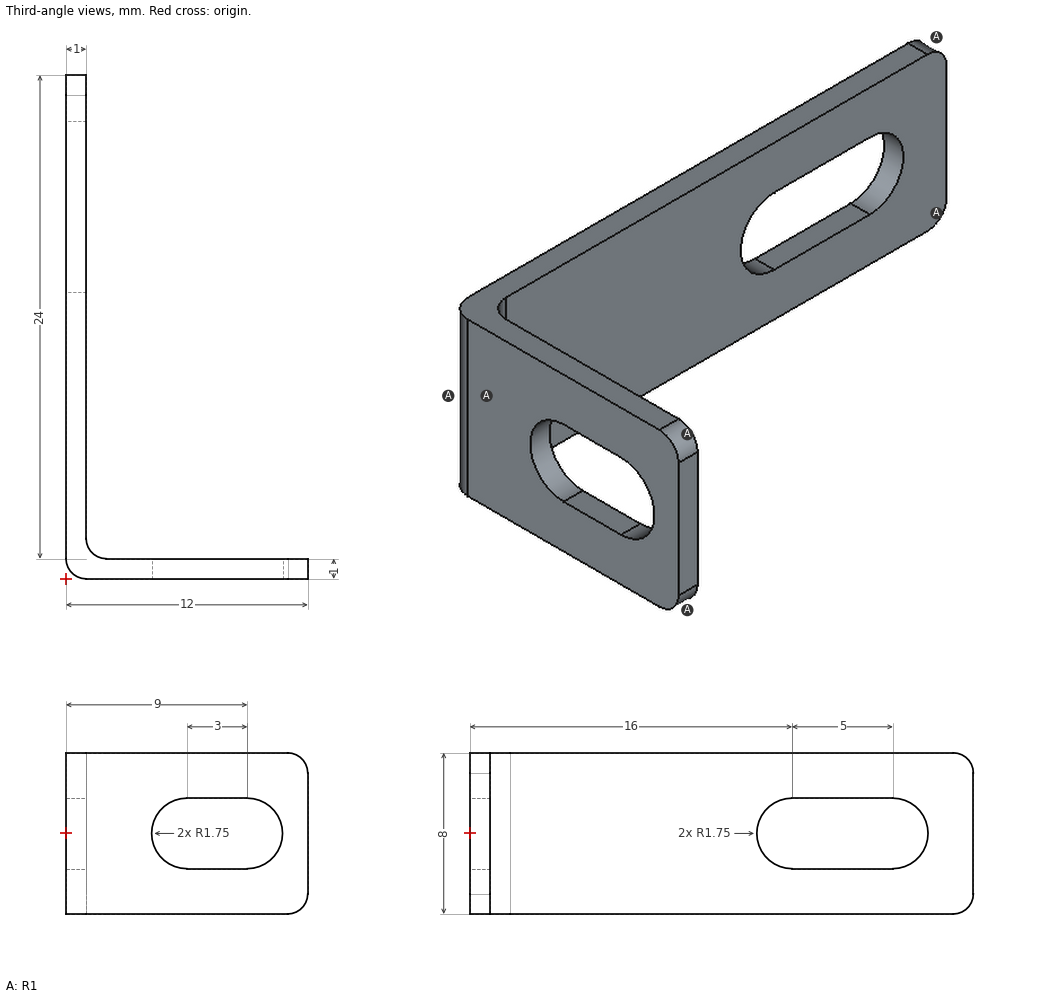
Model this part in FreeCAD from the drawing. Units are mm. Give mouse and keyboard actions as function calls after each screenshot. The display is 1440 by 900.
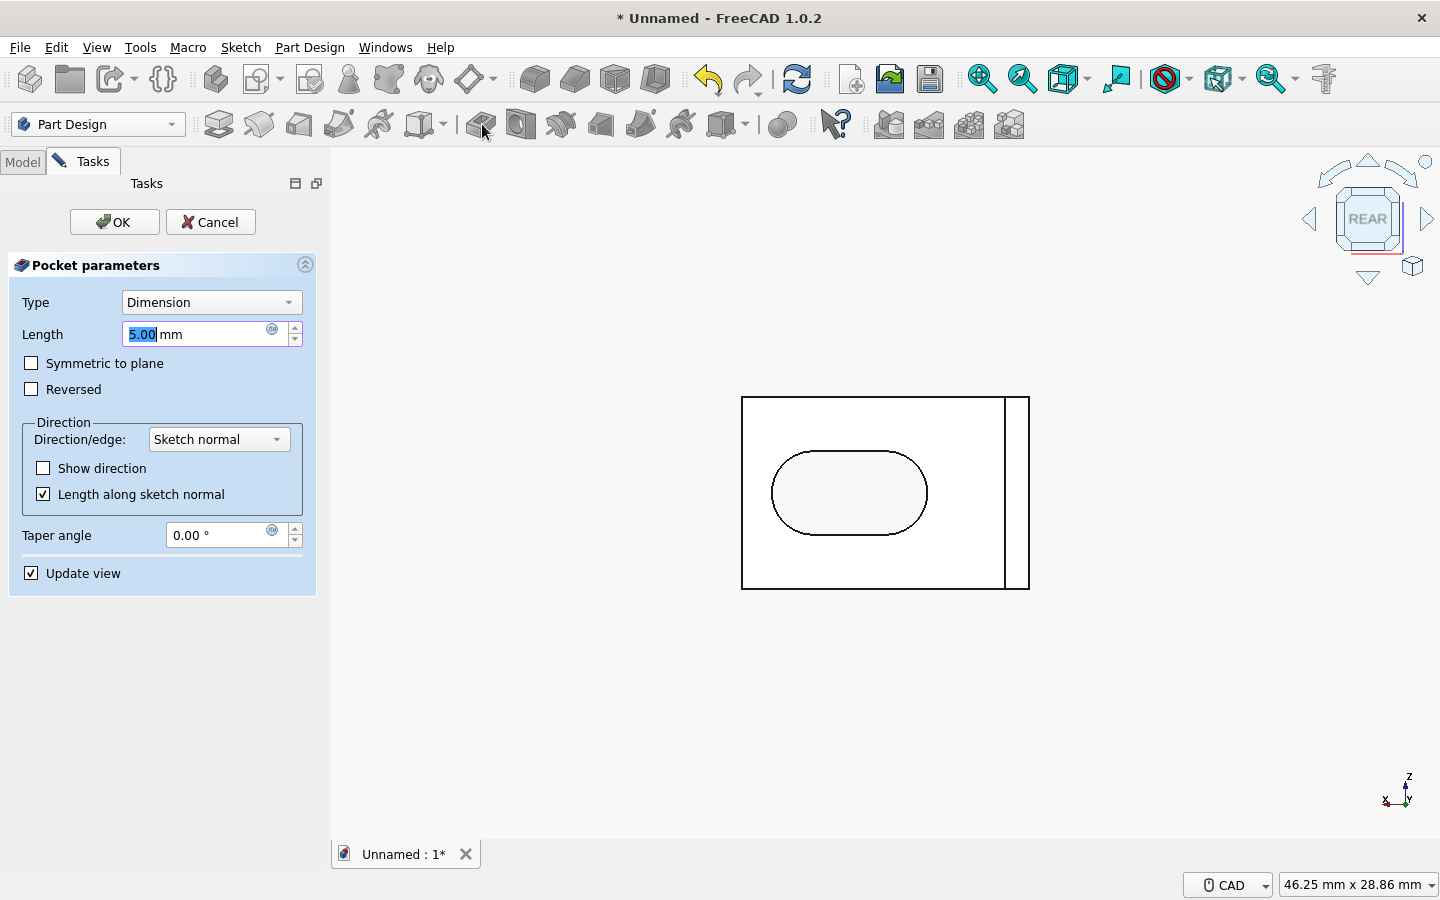
click(212, 302)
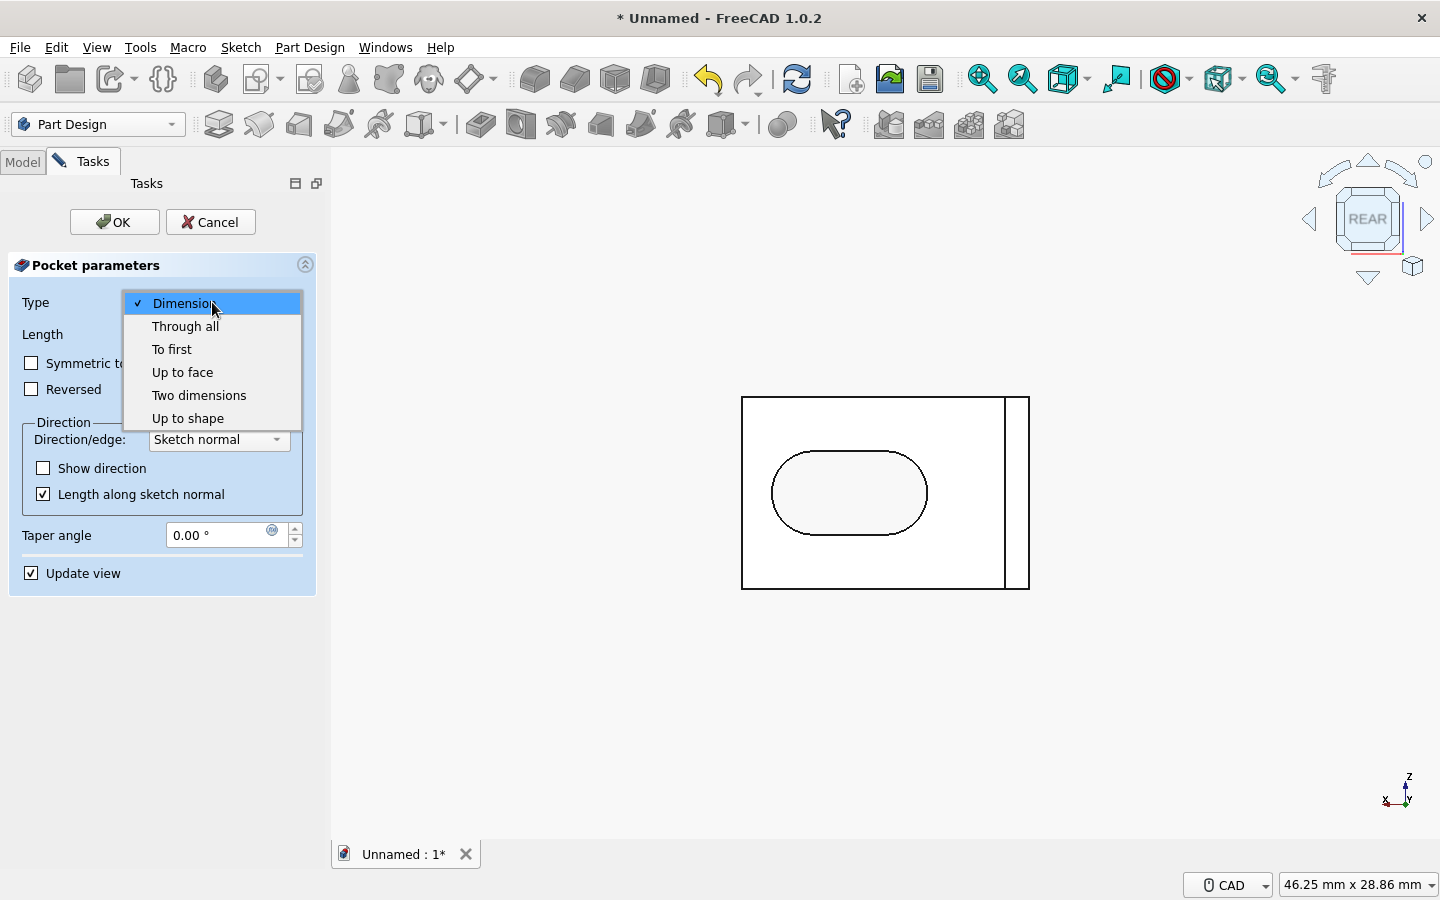
click(212, 326)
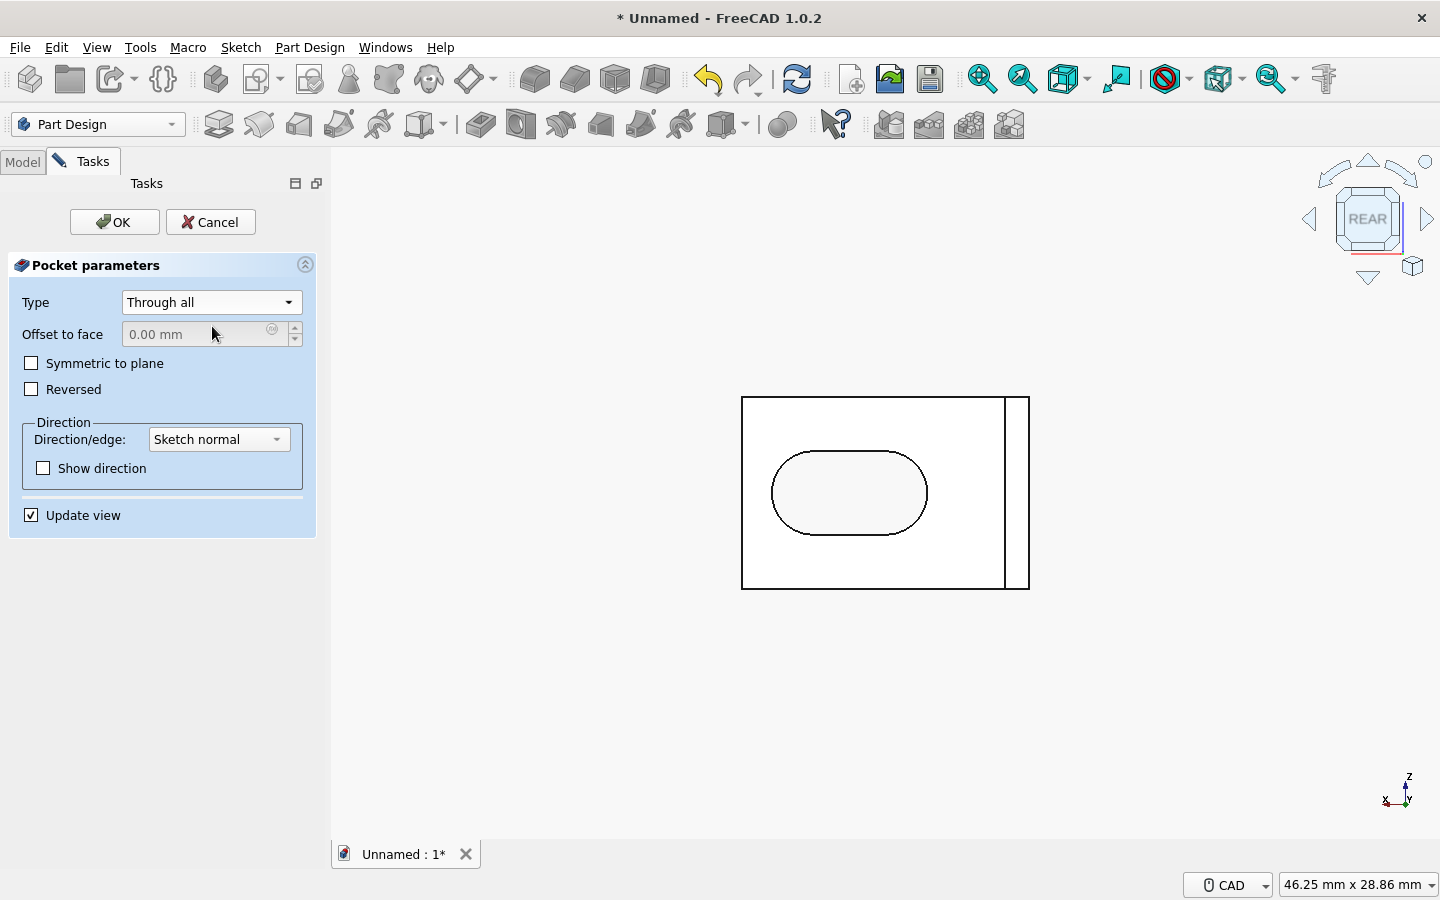
click(30, 389)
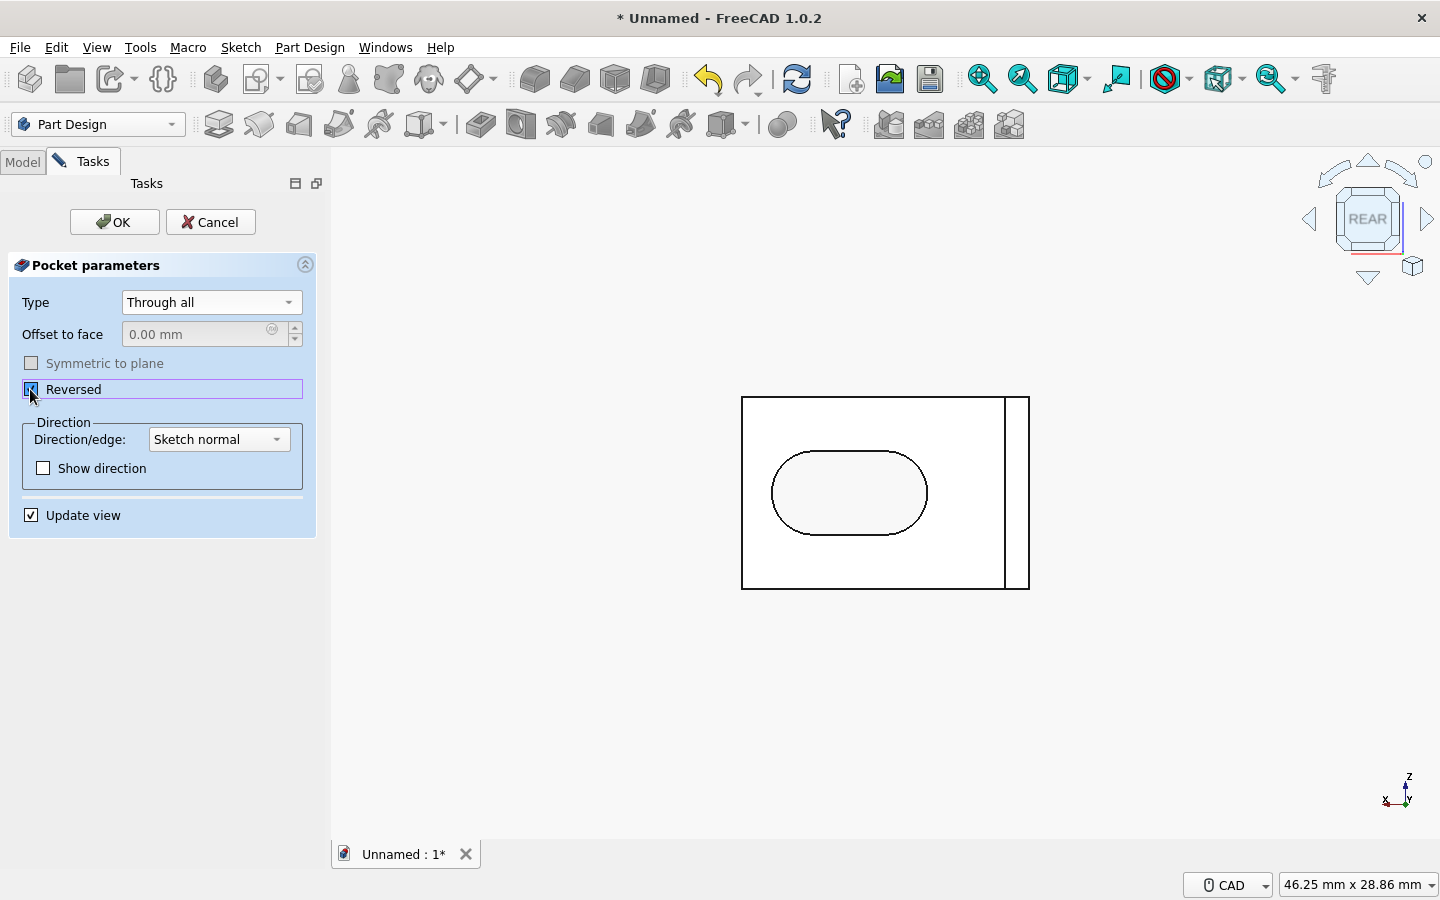
click(115, 222)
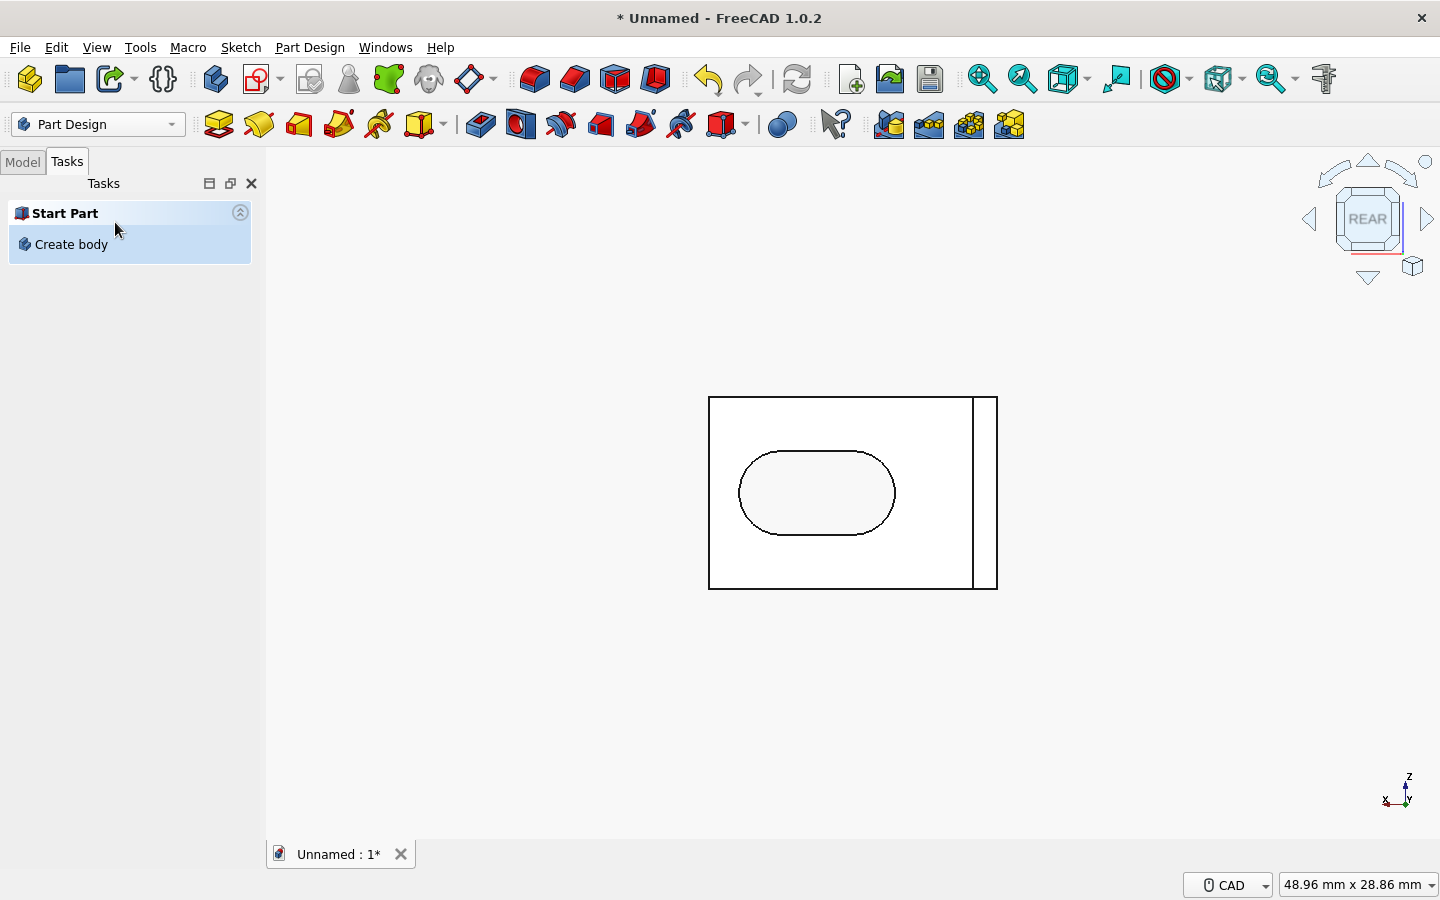
key(v)
key(f)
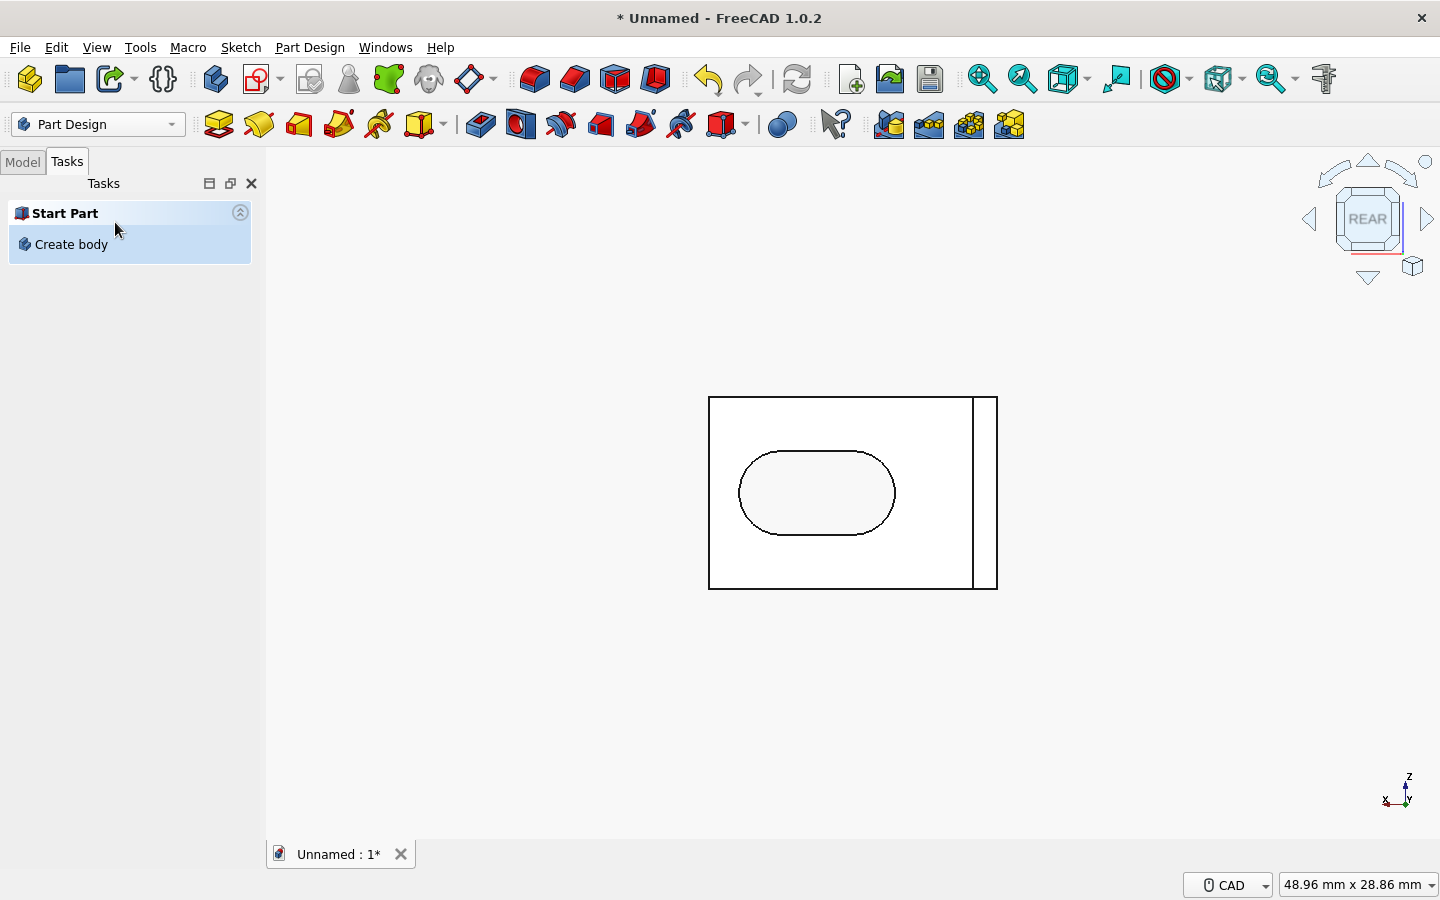
click(985, 396)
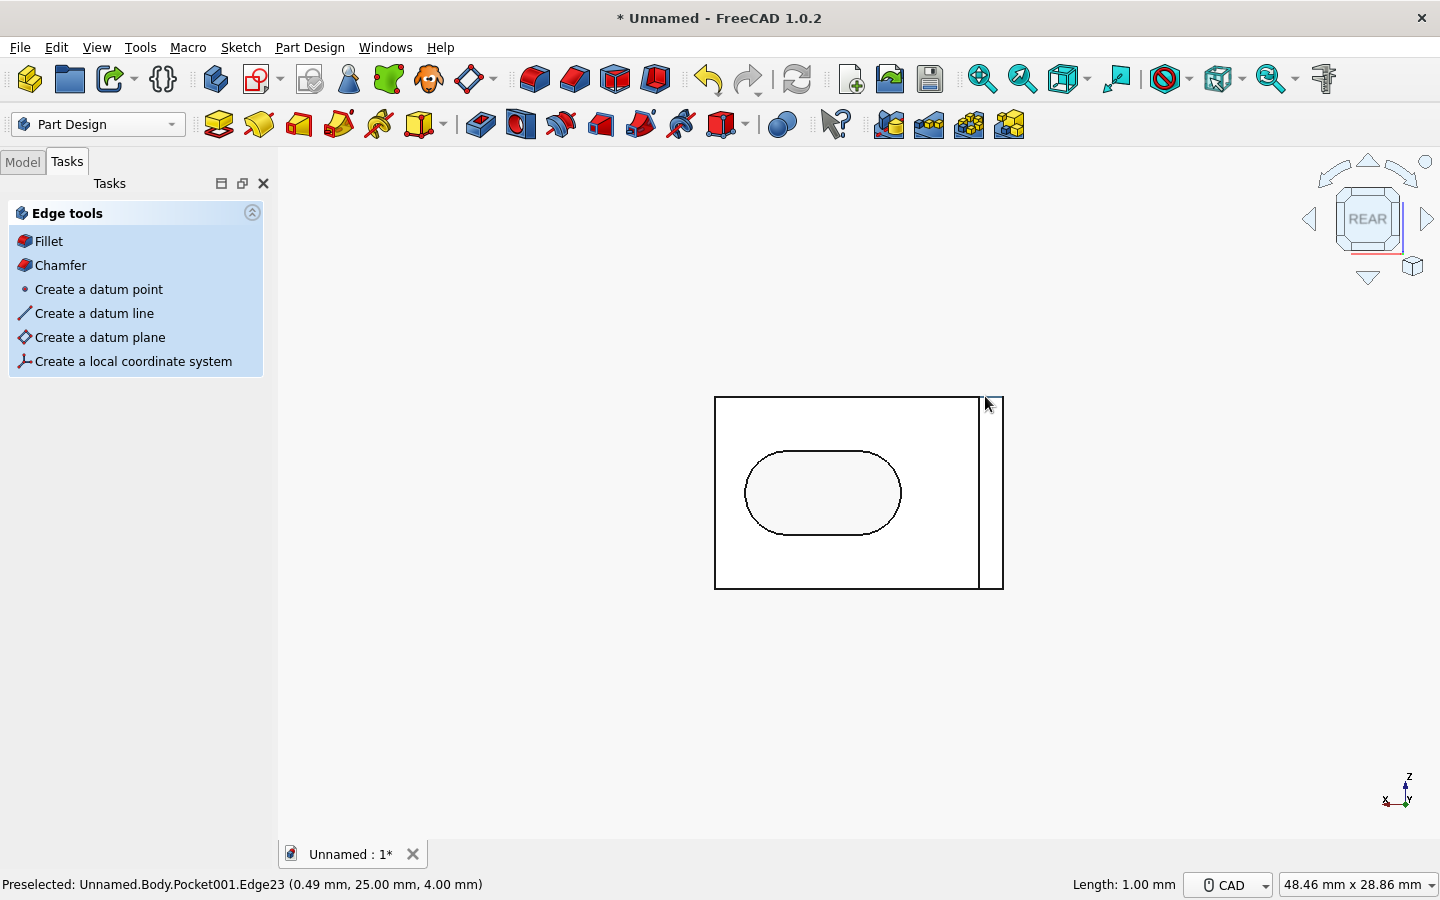
click(991, 588, ctrl)